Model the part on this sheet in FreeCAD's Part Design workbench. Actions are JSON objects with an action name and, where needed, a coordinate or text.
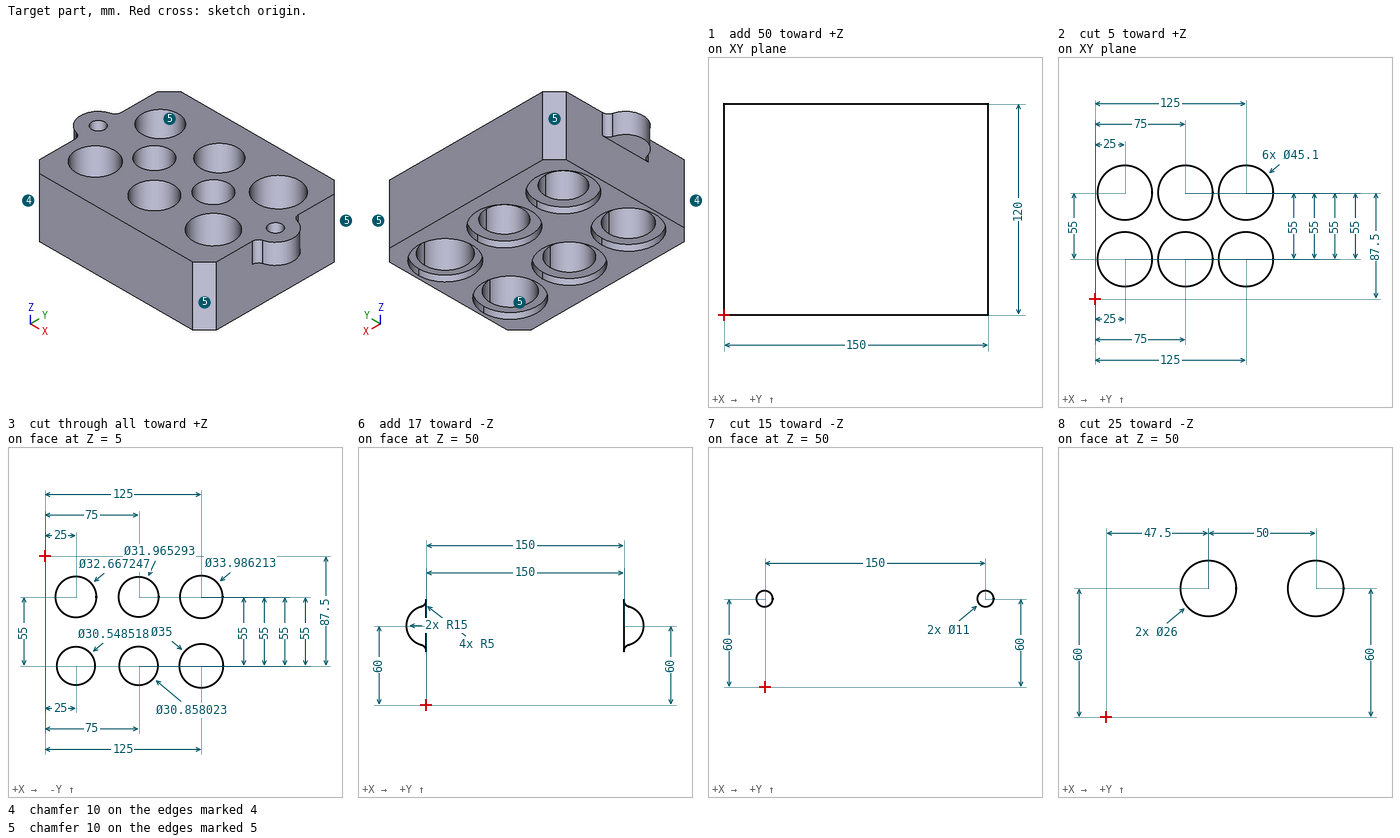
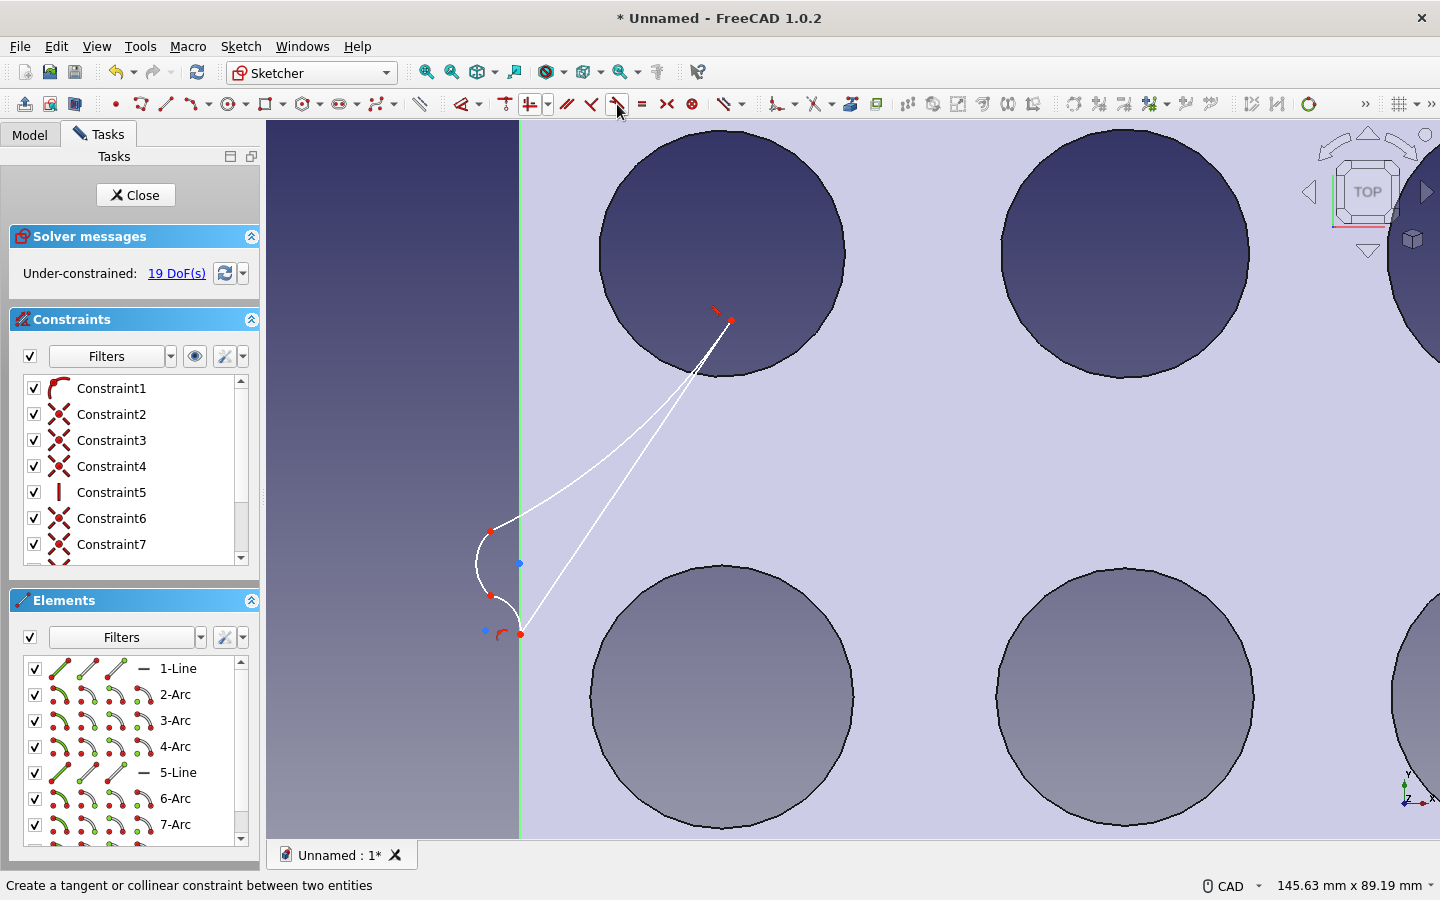
{"action": "left_click", "coordinate": [584, 540]}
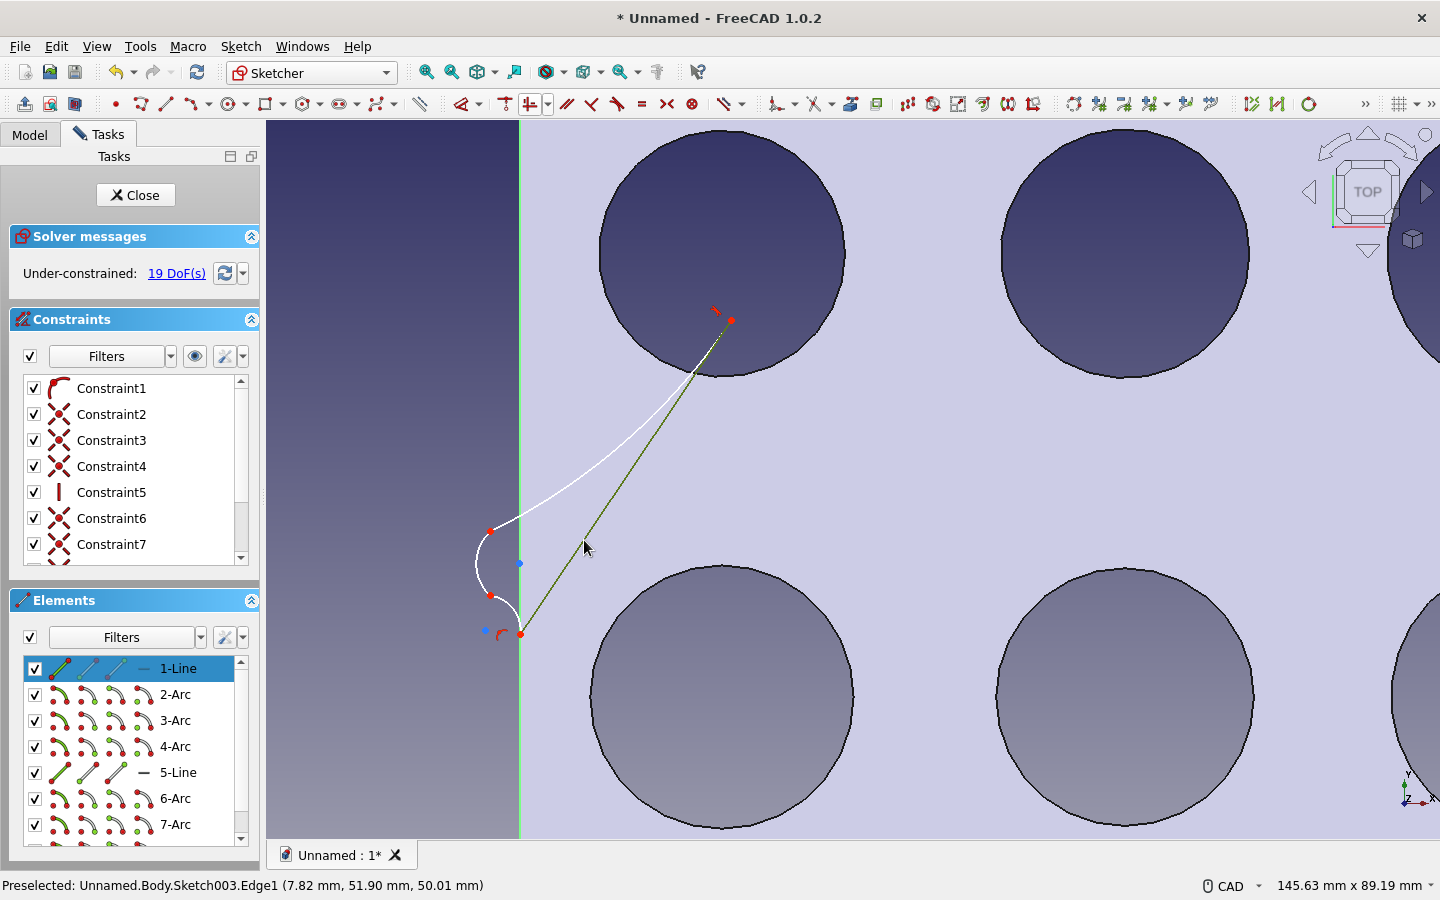
{"action": "scroll", "coordinate": [519, 618], "scroll_direction": "up", "scroll_amount": 2}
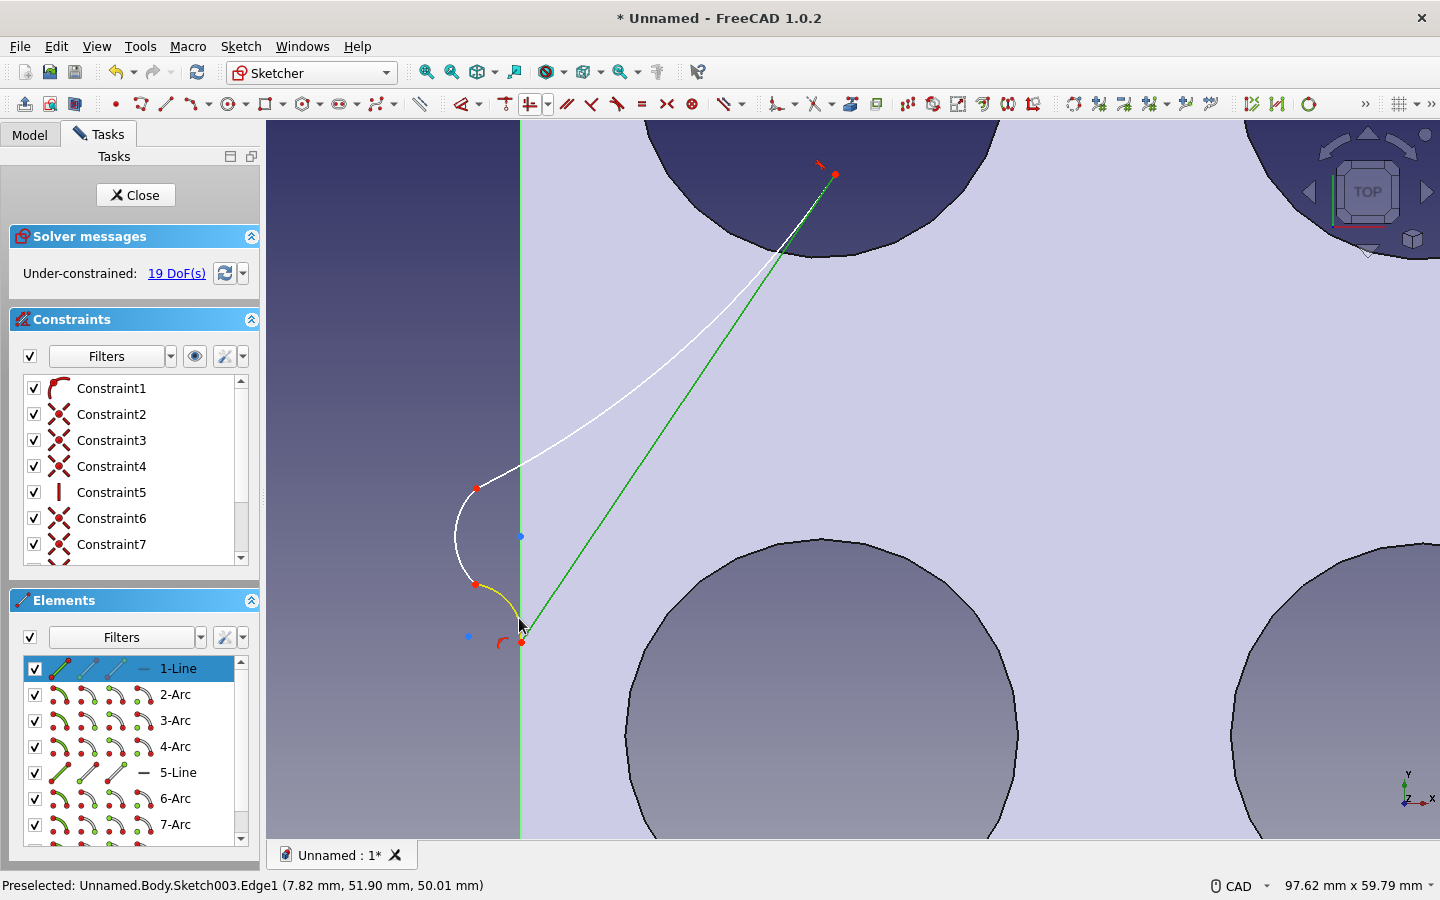
{"action": "left_click", "coordinate": [518, 618]}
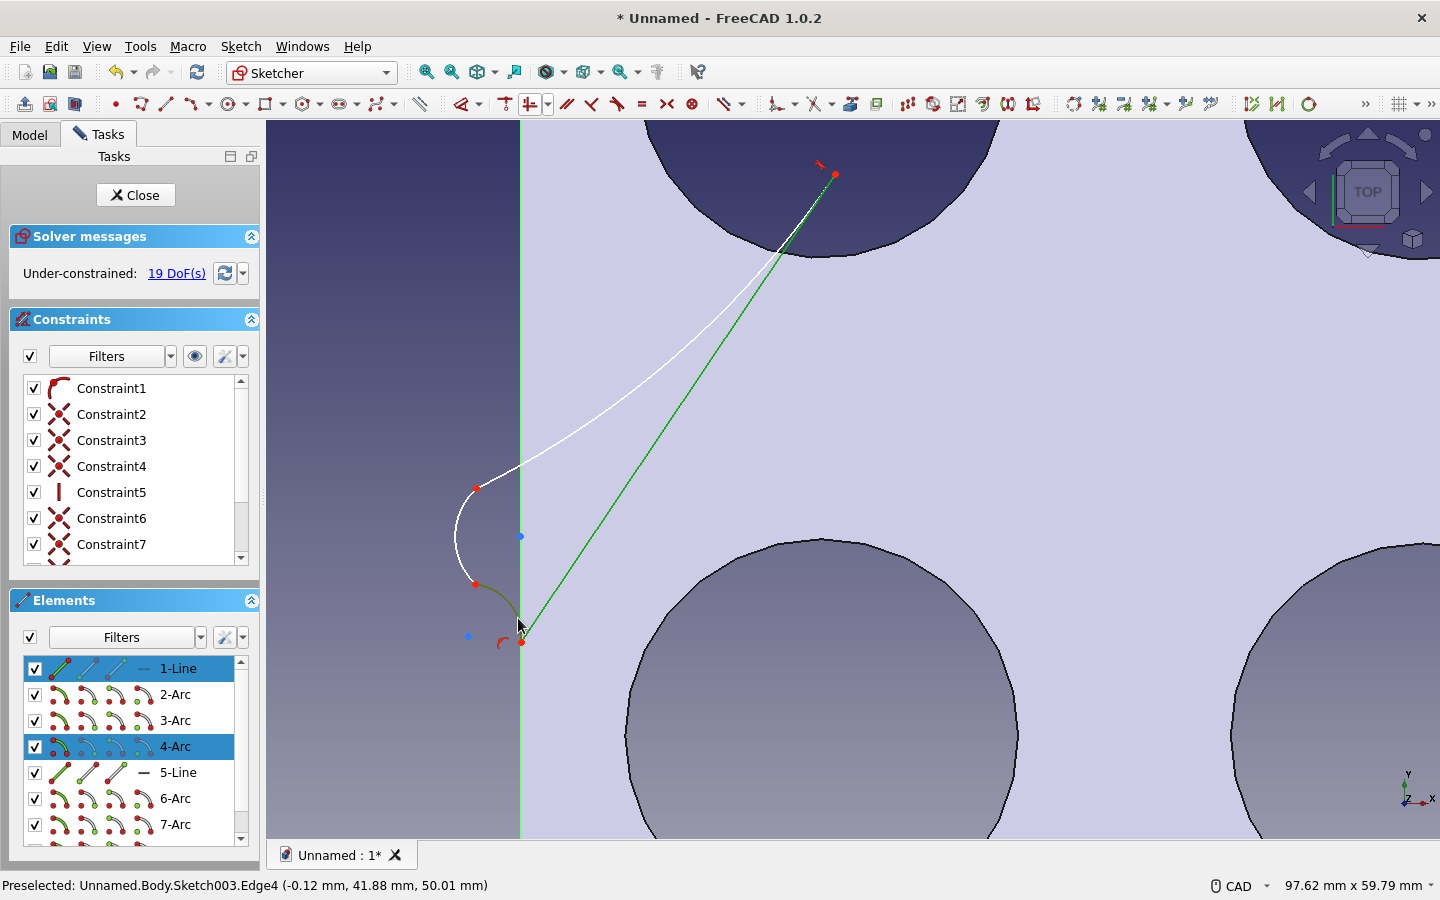
{"action": "key", "text": "t"}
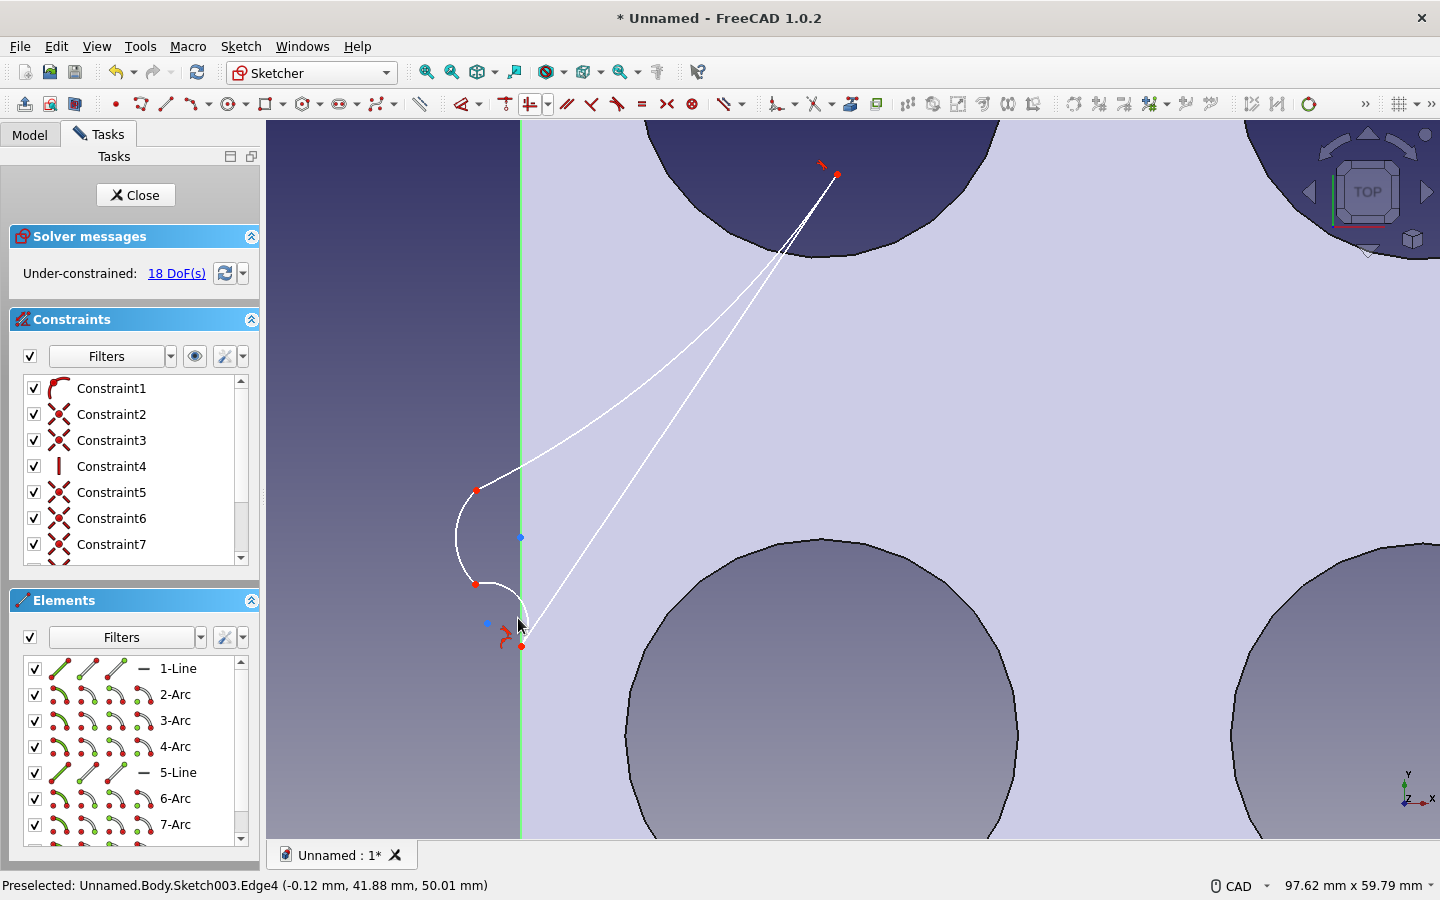
{"action": "left_click", "coordinate": [602, 416]}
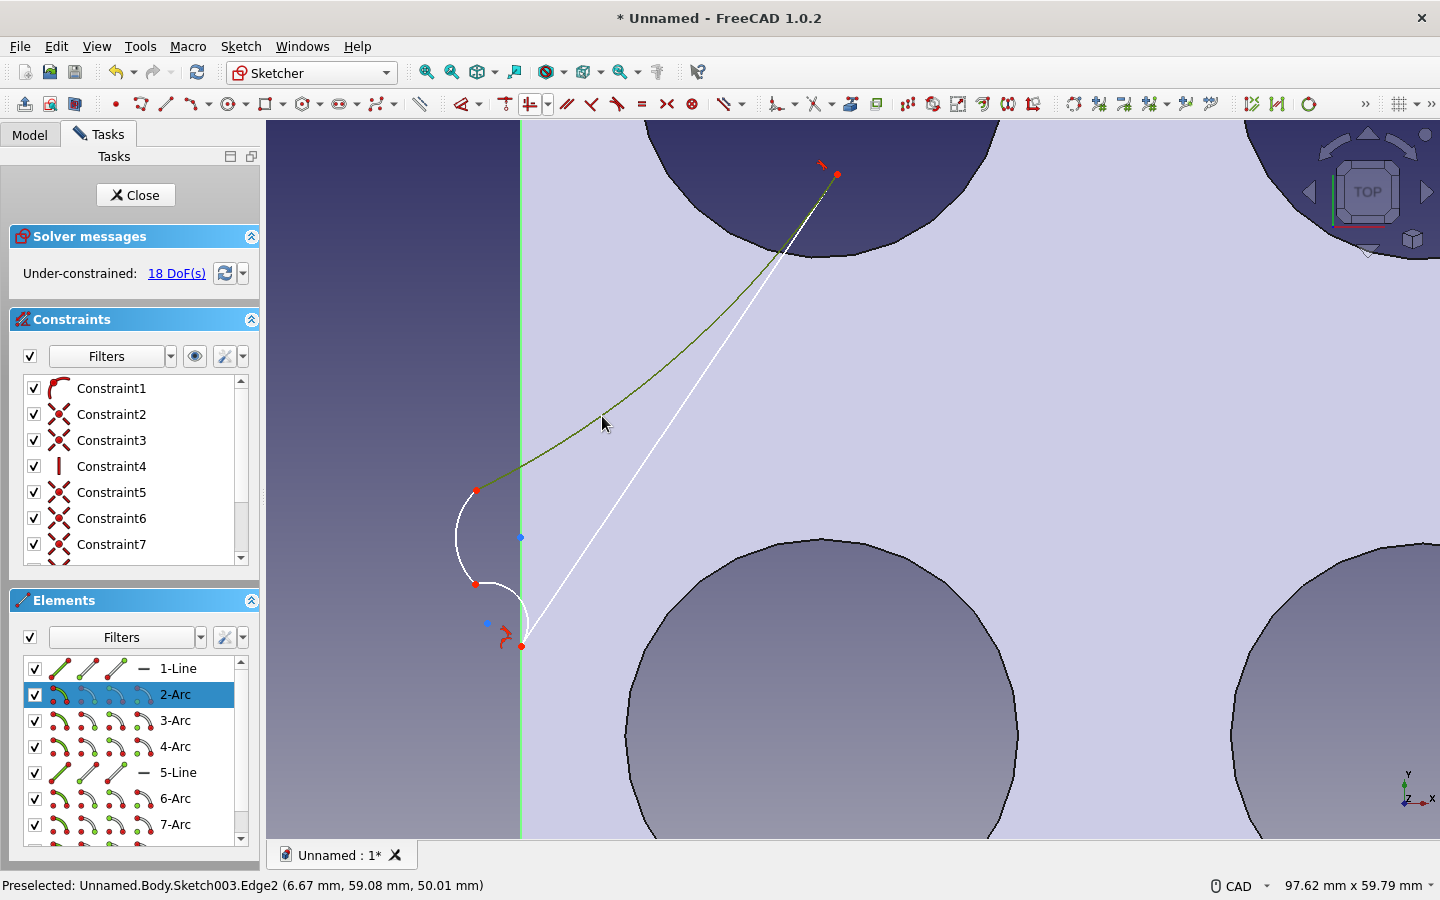
{"action": "left_click", "coordinate": [459, 516]}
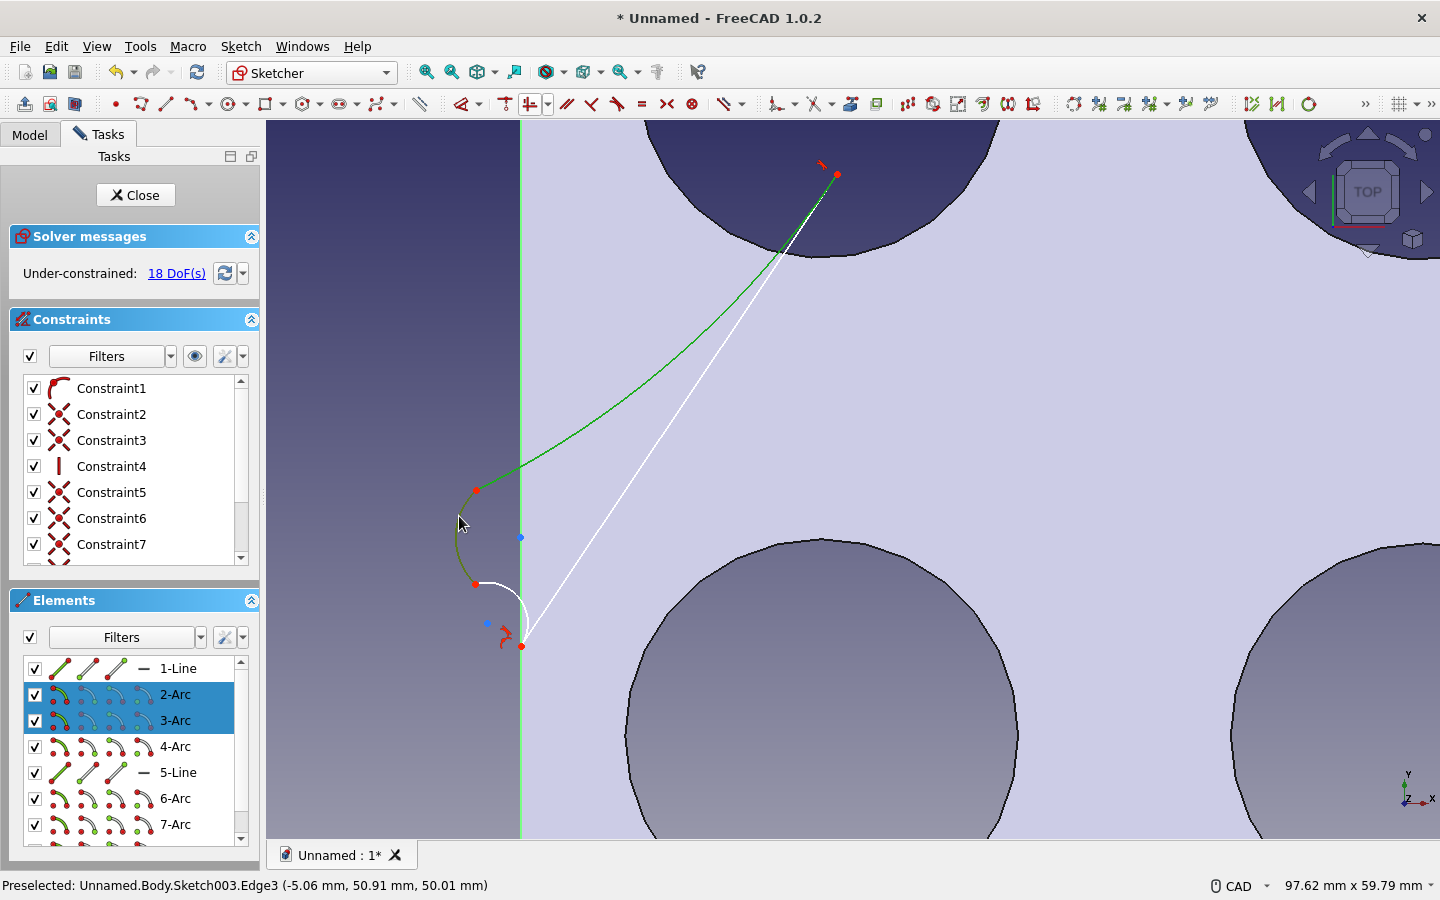
{"action": "key", "text": "t"}